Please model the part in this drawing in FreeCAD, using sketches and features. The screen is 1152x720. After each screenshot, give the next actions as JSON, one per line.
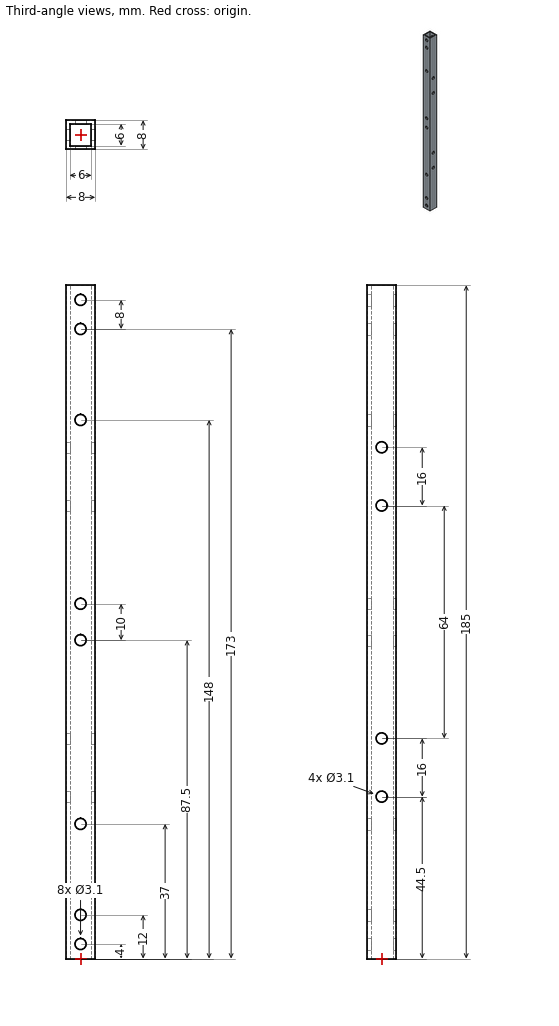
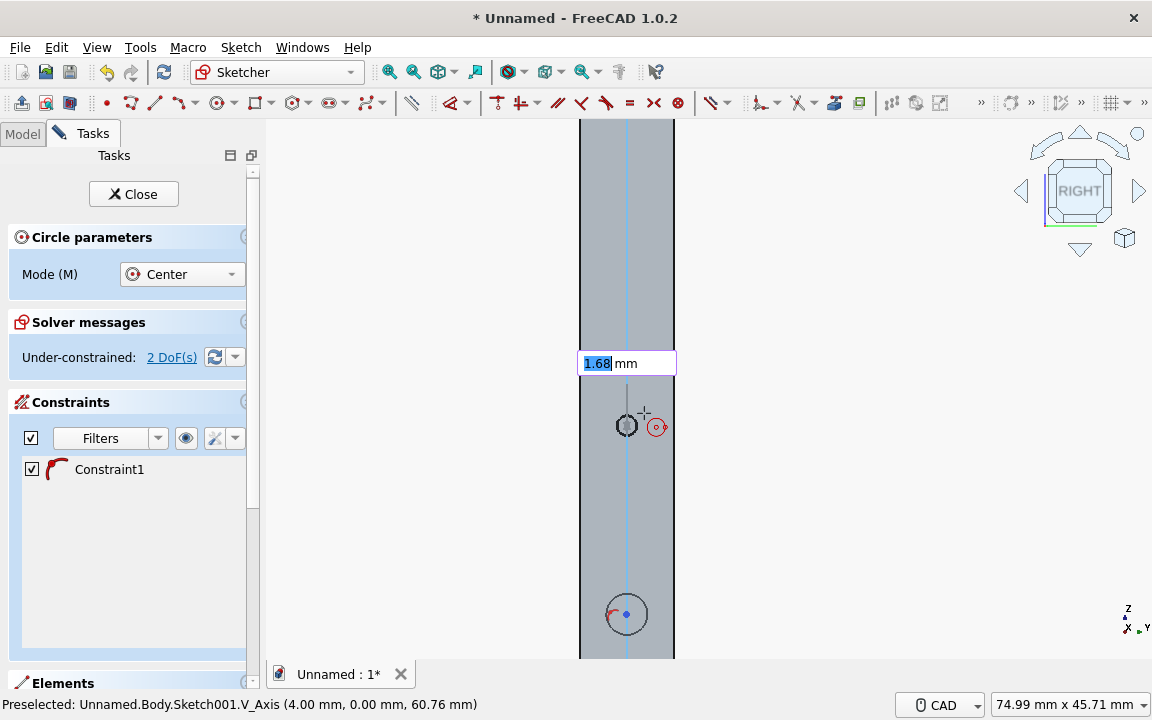
{"action": "left_click", "coordinate": [644, 413]}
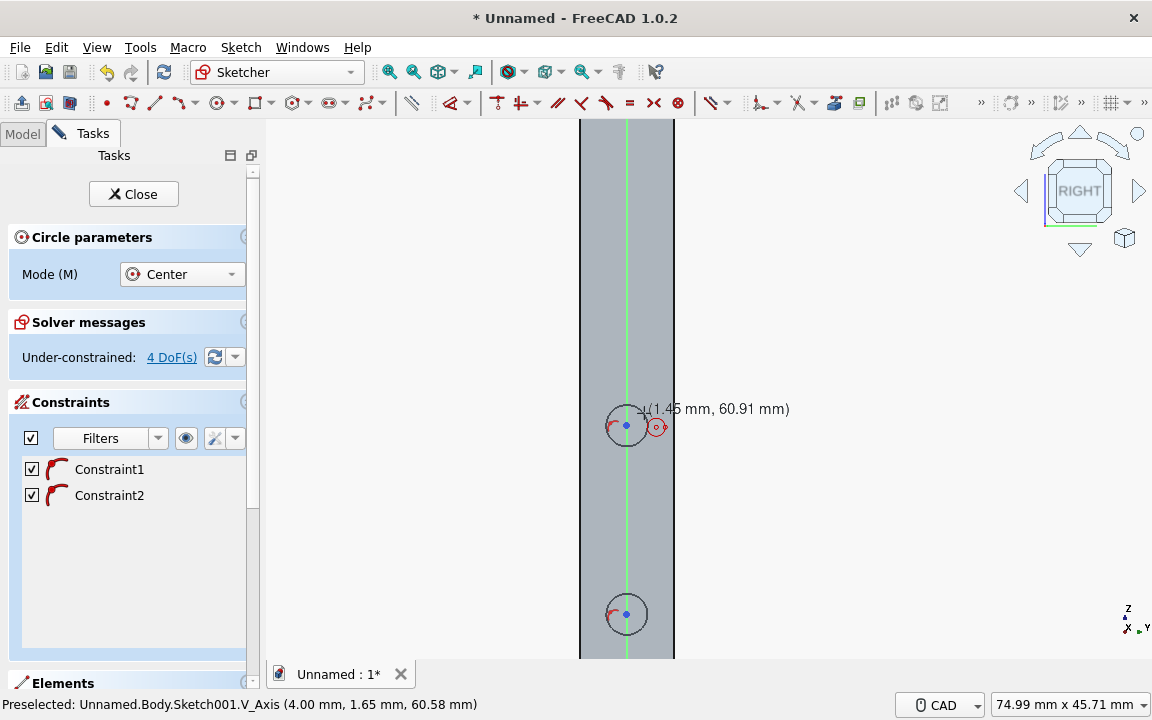
{"action": "scroll", "coordinate": [644, 413], "scroll_direction": "down", "scroll_amount": 8}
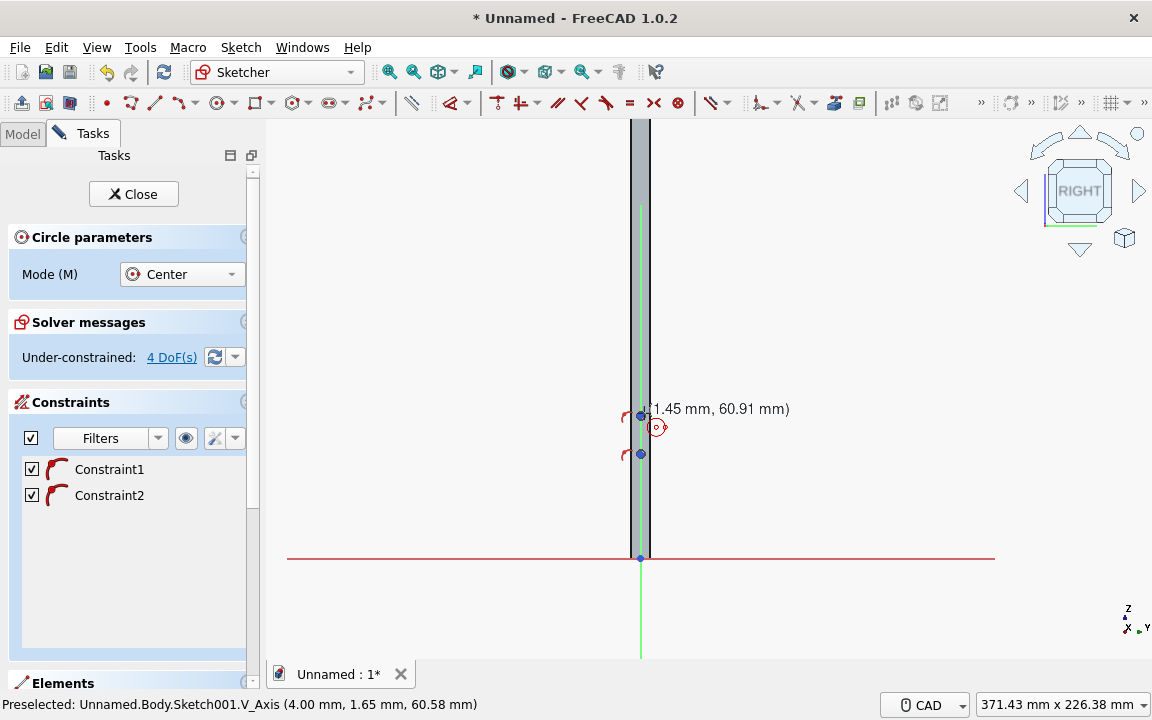
{"action": "scroll", "coordinate": [641, 262], "scroll_direction": "up", "scroll_amount": 10}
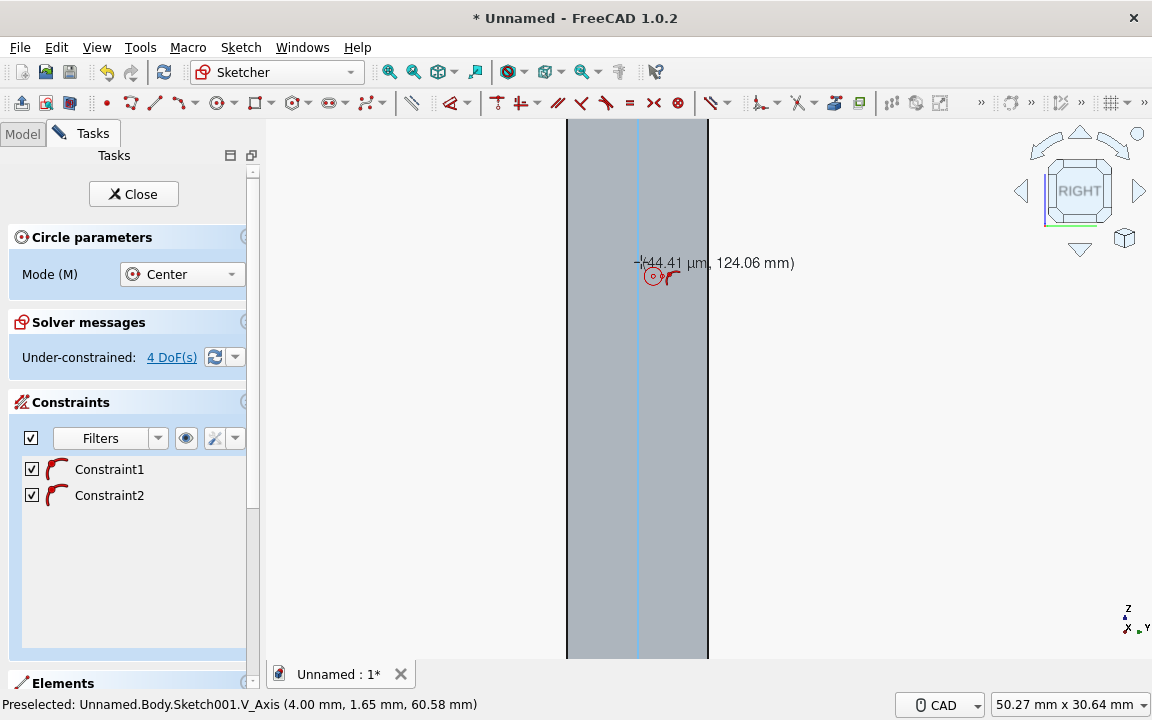
{"action": "scroll", "coordinate": [641, 262], "scroll_direction": "down", "scroll_amount": 10}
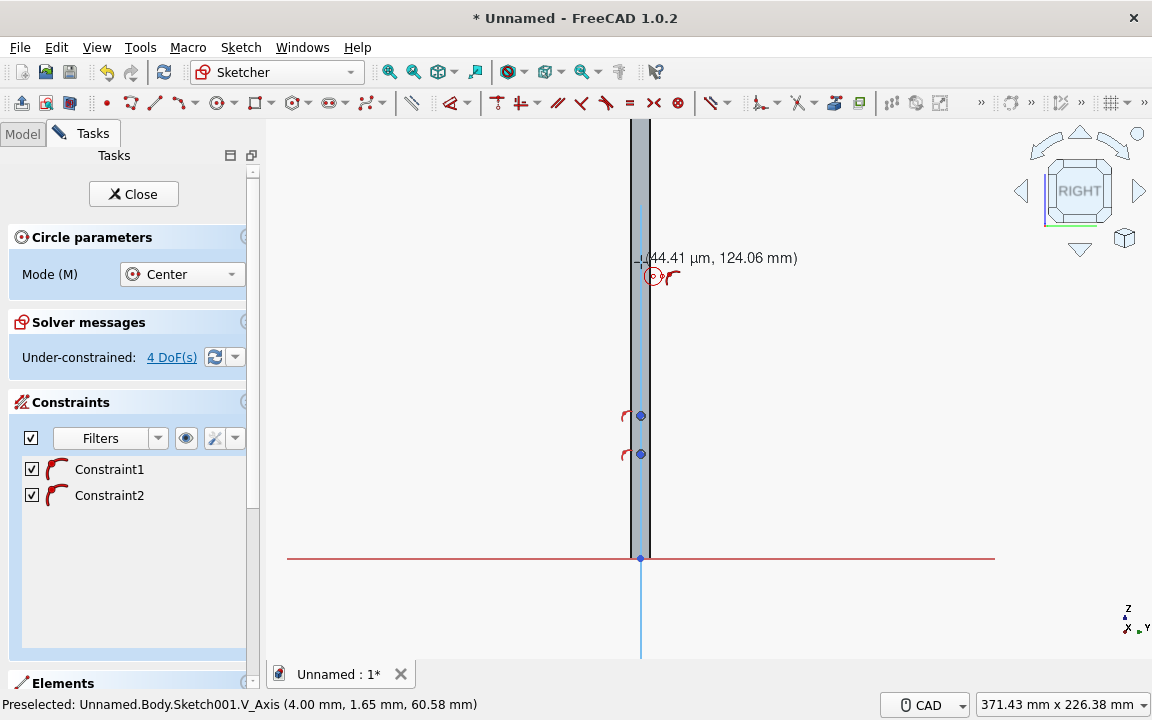
{"action": "left_click", "coordinate": [641, 262]}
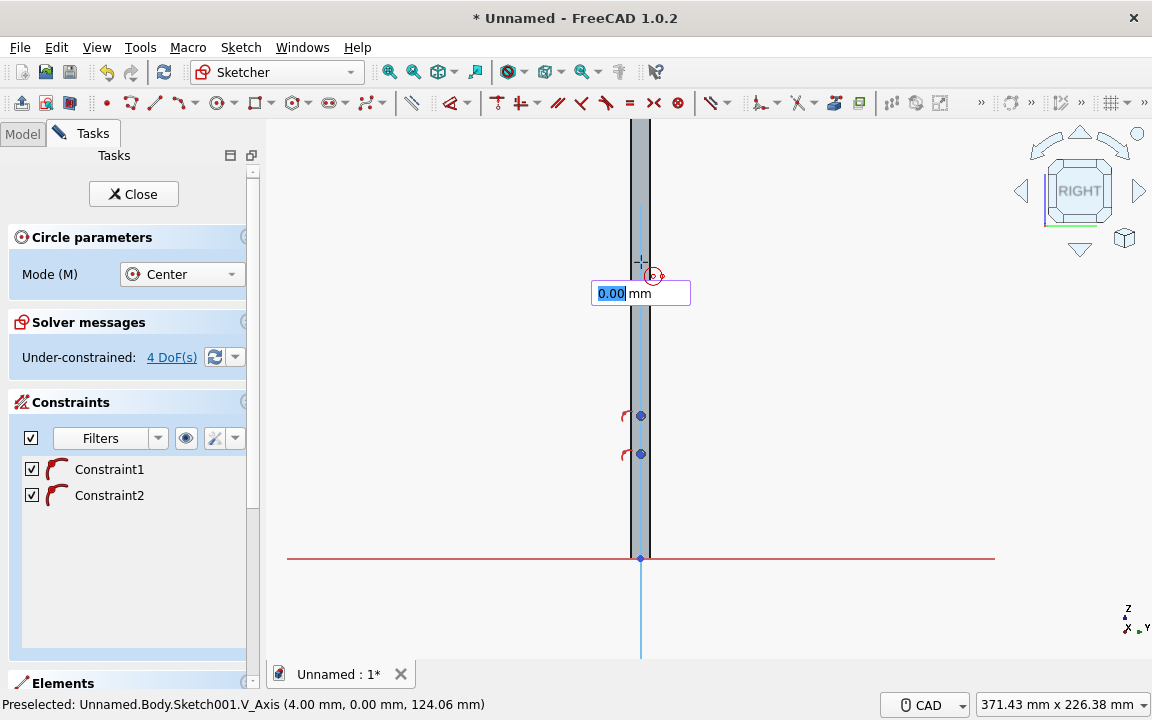
{"action": "scroll", "coordinate": [644, 261], "scroll_direction": "up", "scroll_amount": 8}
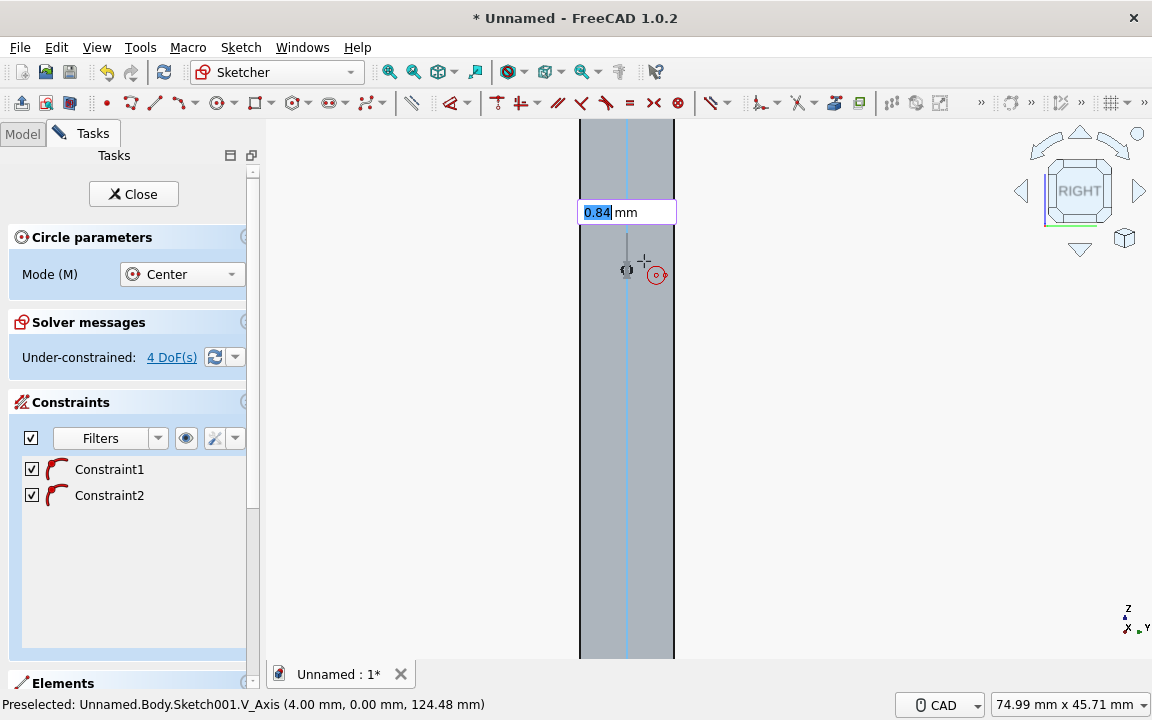
{"action": "left_click", "coordinate": [644, 258]}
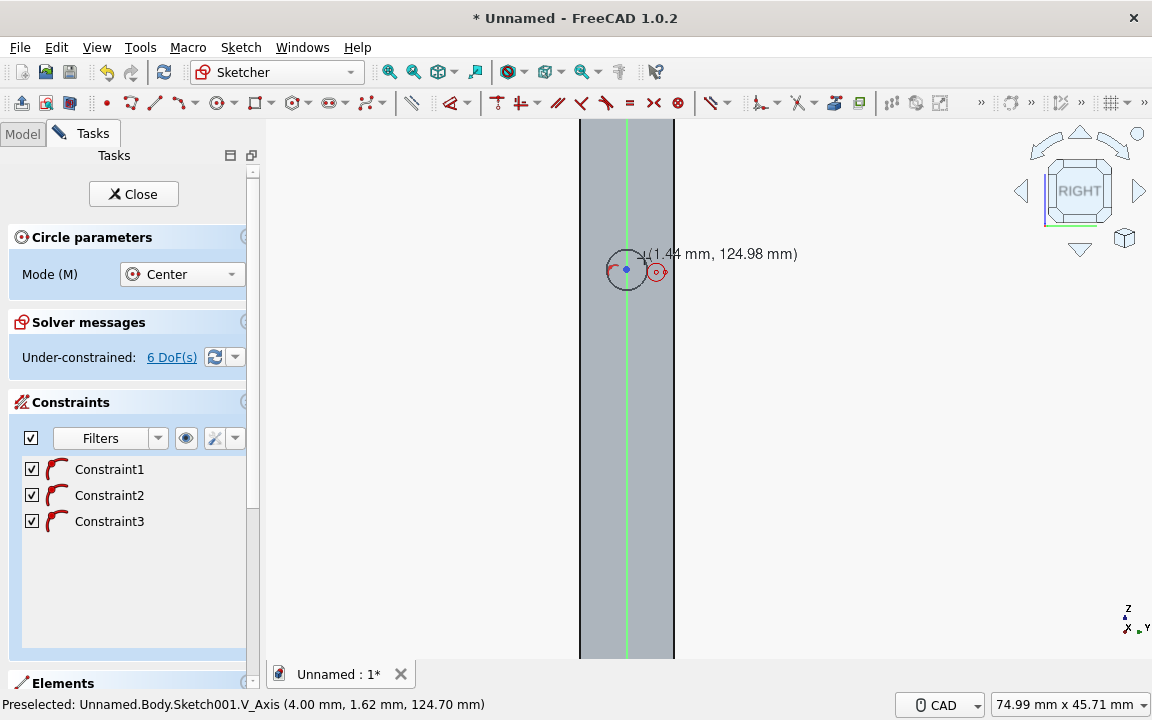
{"action": "scroll", "coordinate": [644, 261], "scroll_direction": "down", "scroll_amount": 8}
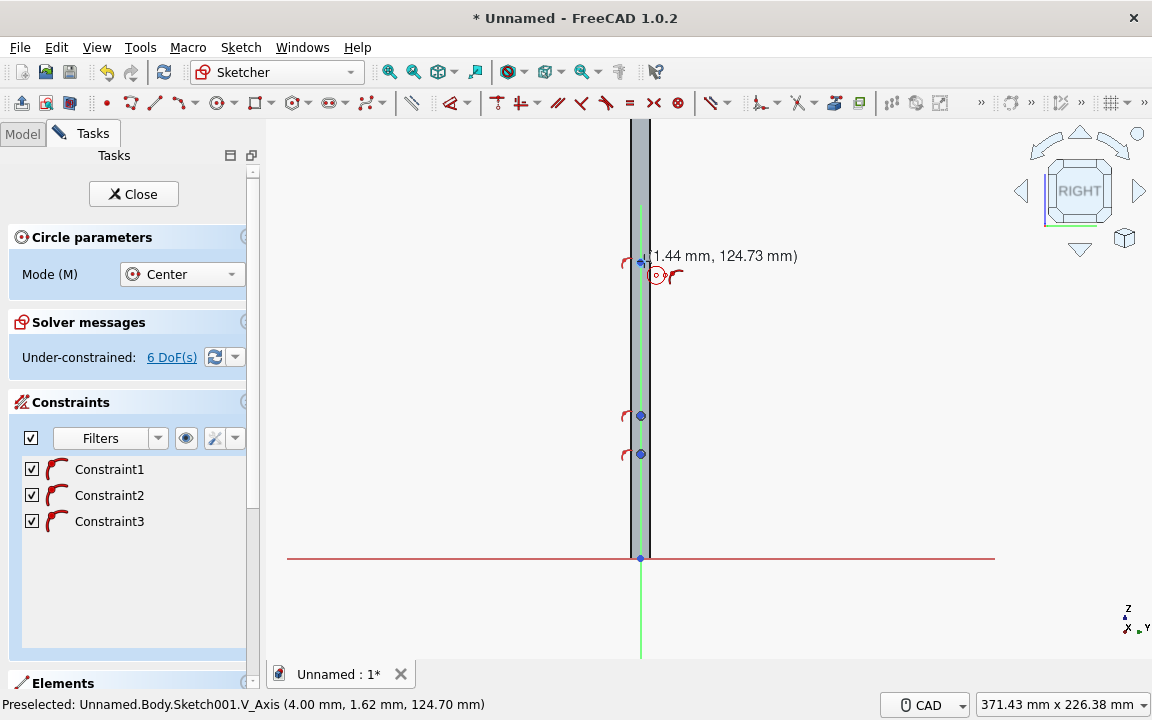
{"action": "scroll", "coordinate": [641, 224], "scroll_direction": "up", "scroll_amount": 10}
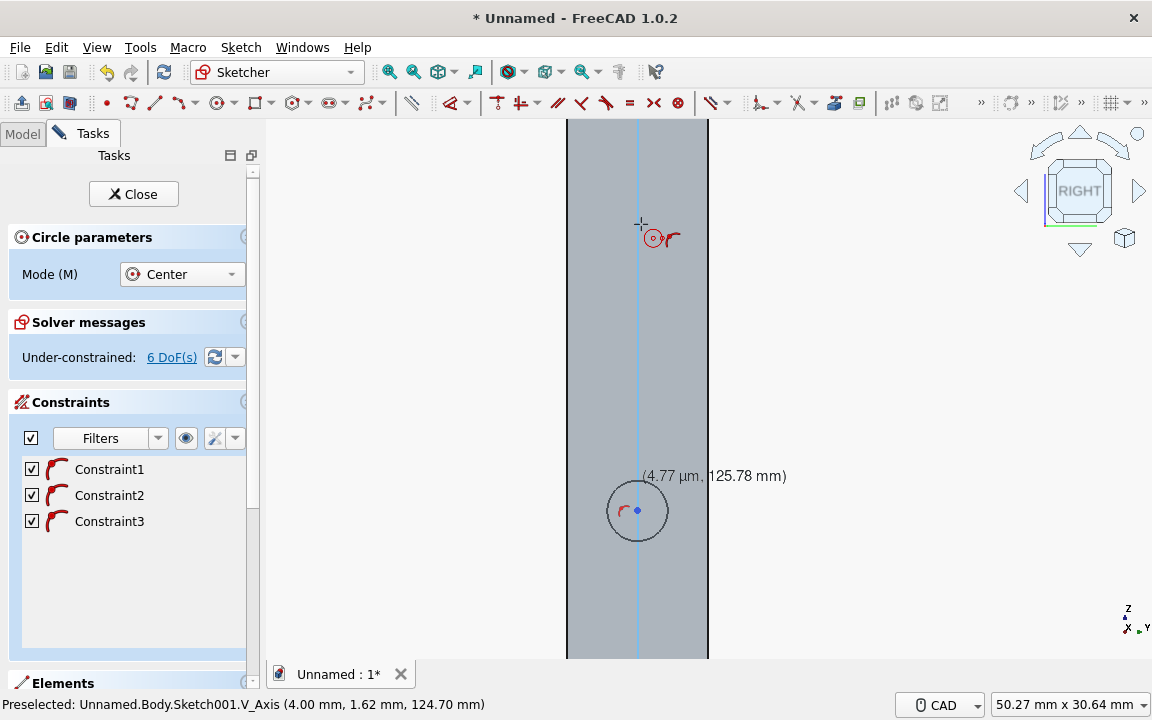
{"action": "scroll", "coordinate": [641, 224], "scroll_direction": "down", "scroll_amount": 10}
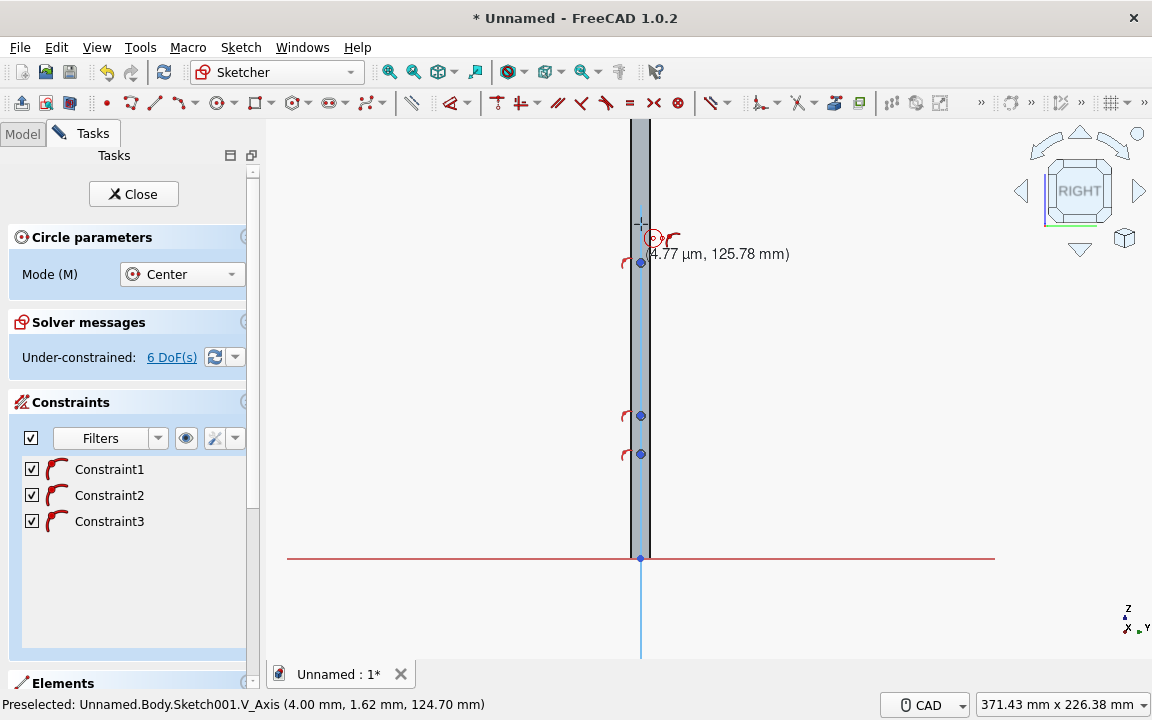
{"action": "left_click", "coordinate": [641, 224]}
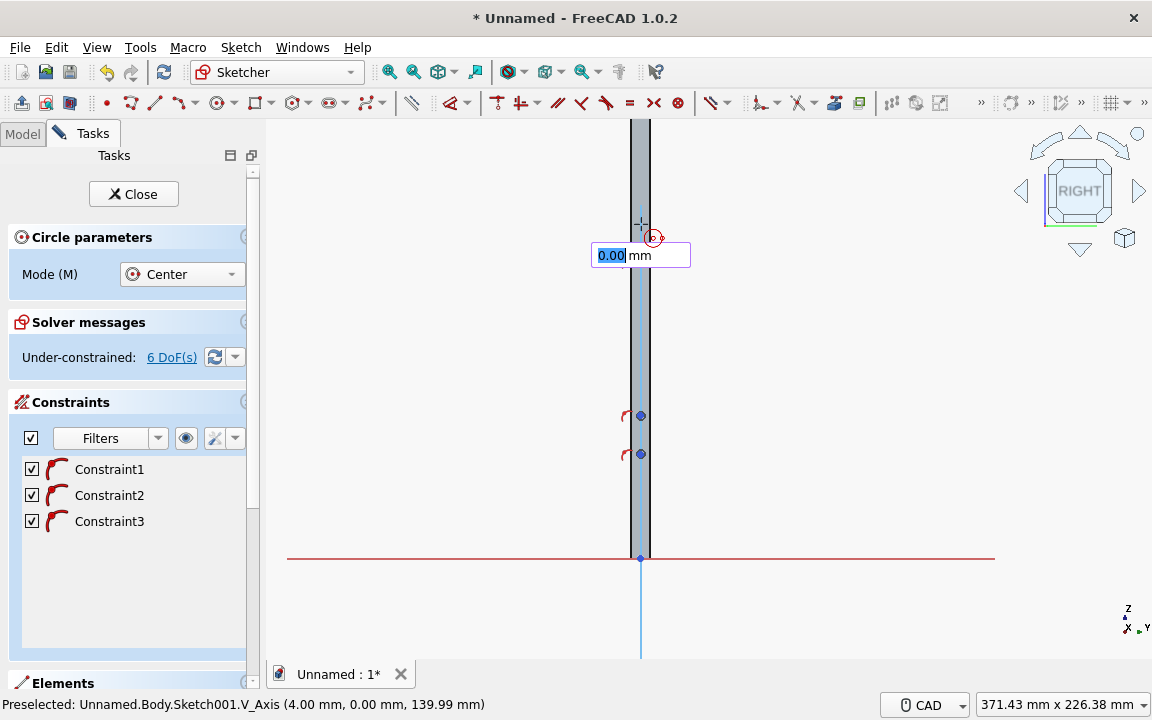
{"action": "scroll", "coordinate": [644, 223], "scroll_direction": "up", "scroll_amount": 8}